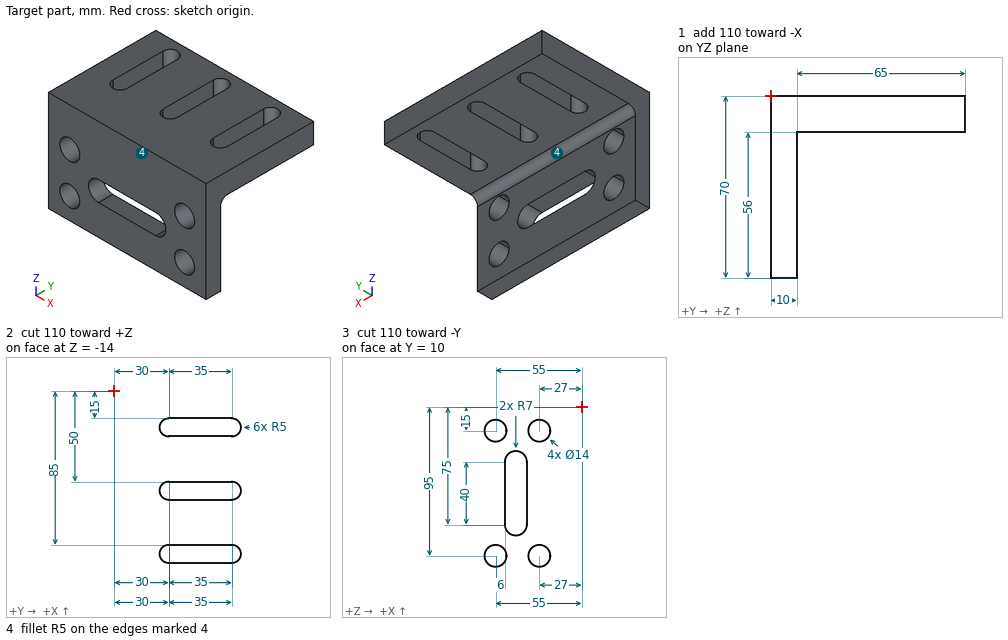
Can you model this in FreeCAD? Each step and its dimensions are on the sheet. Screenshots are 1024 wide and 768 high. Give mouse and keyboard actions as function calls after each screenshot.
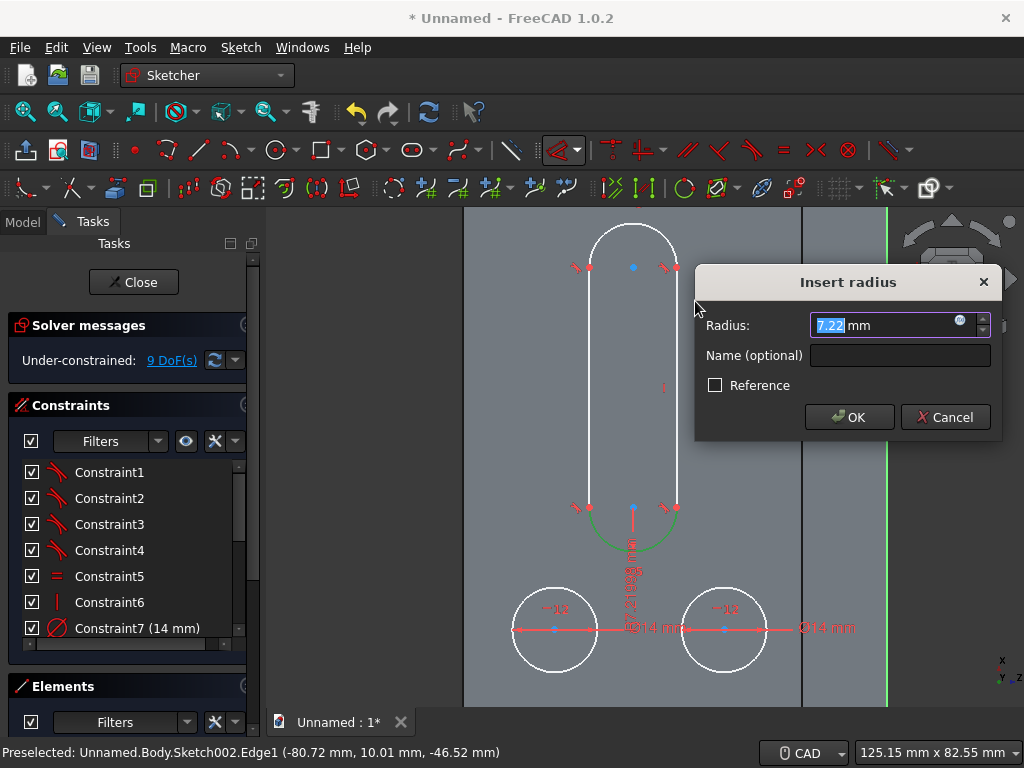
text(7)
key(Return)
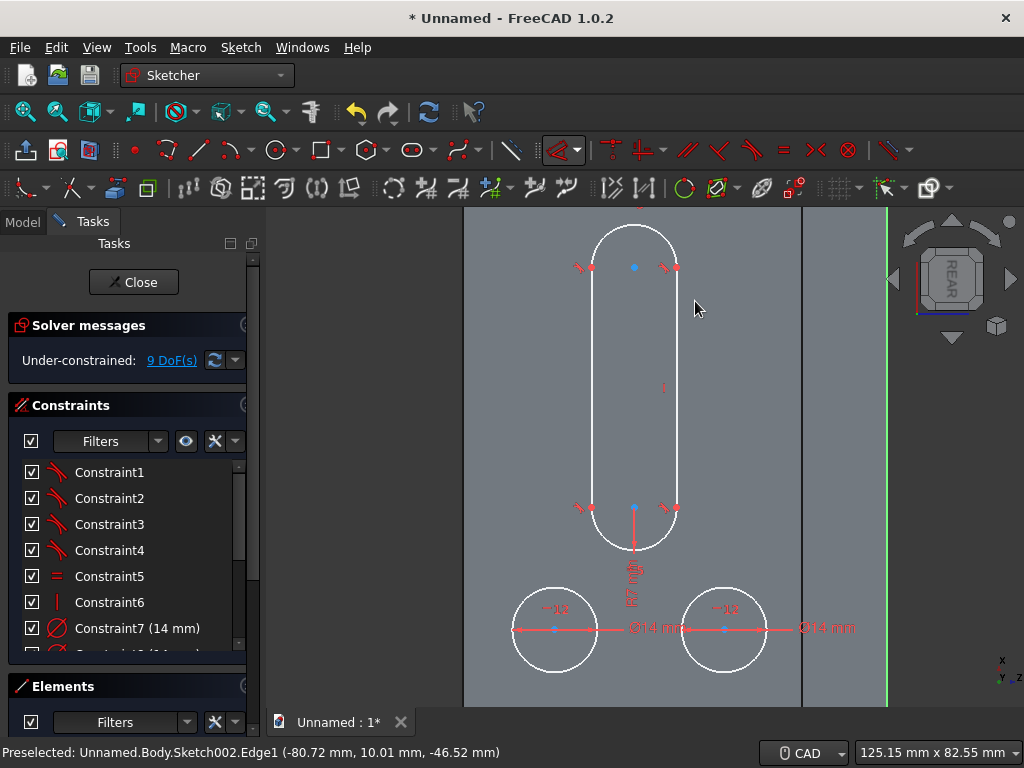
click(592, 436)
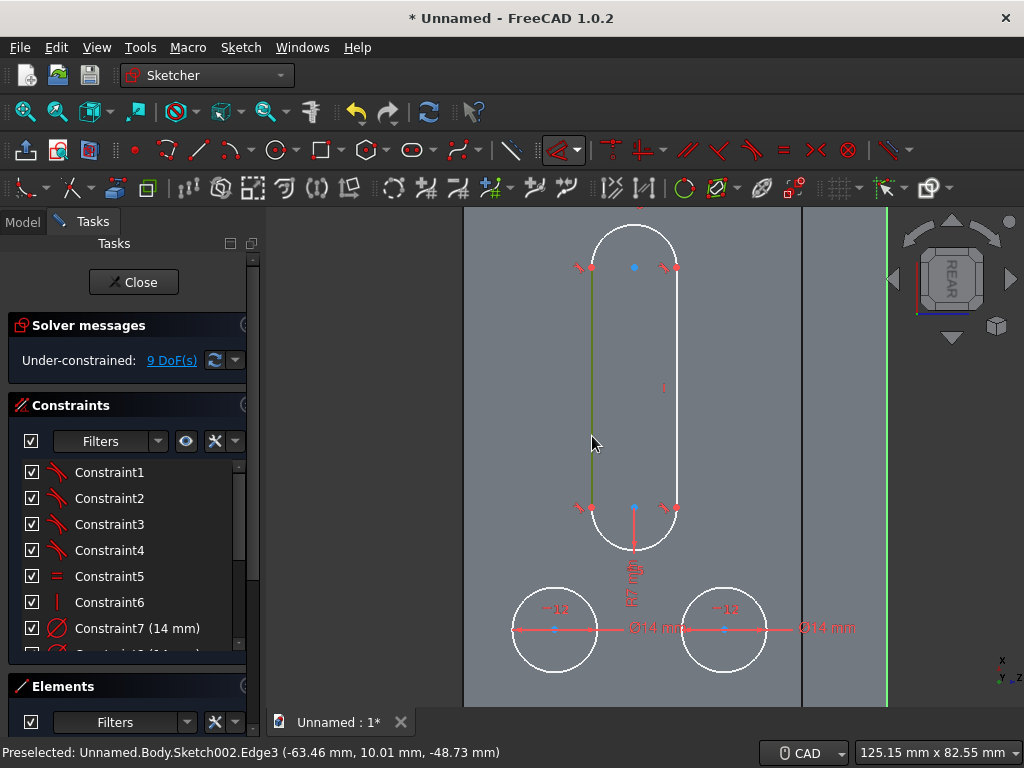
key(i)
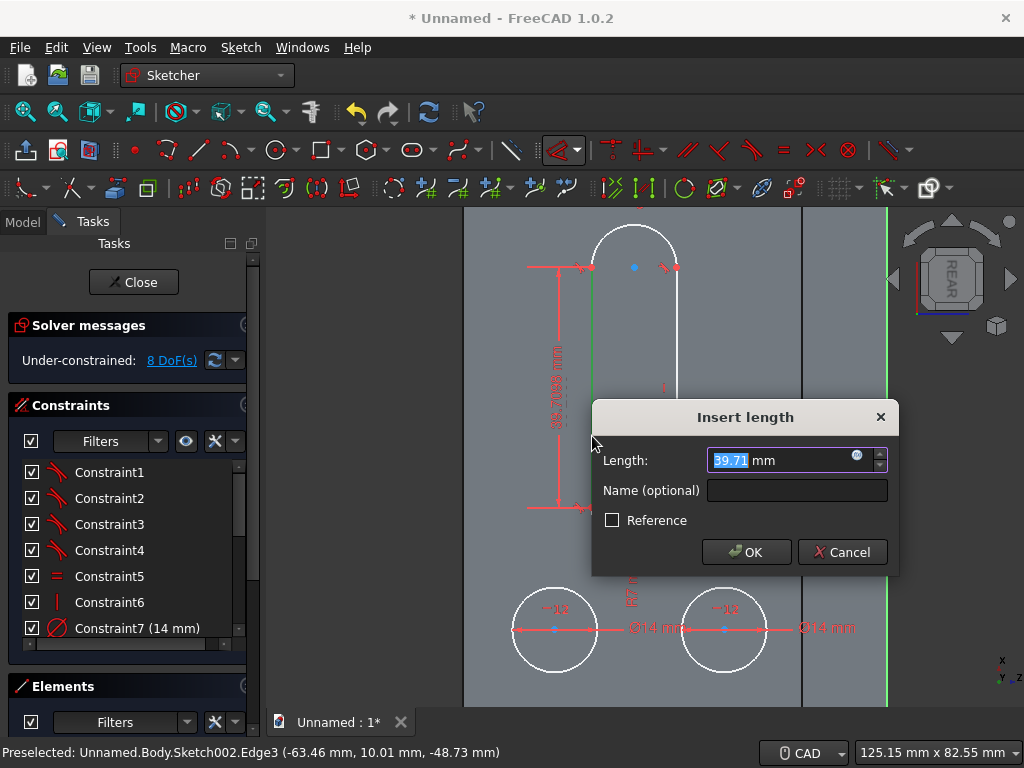
text(40)
key(Return)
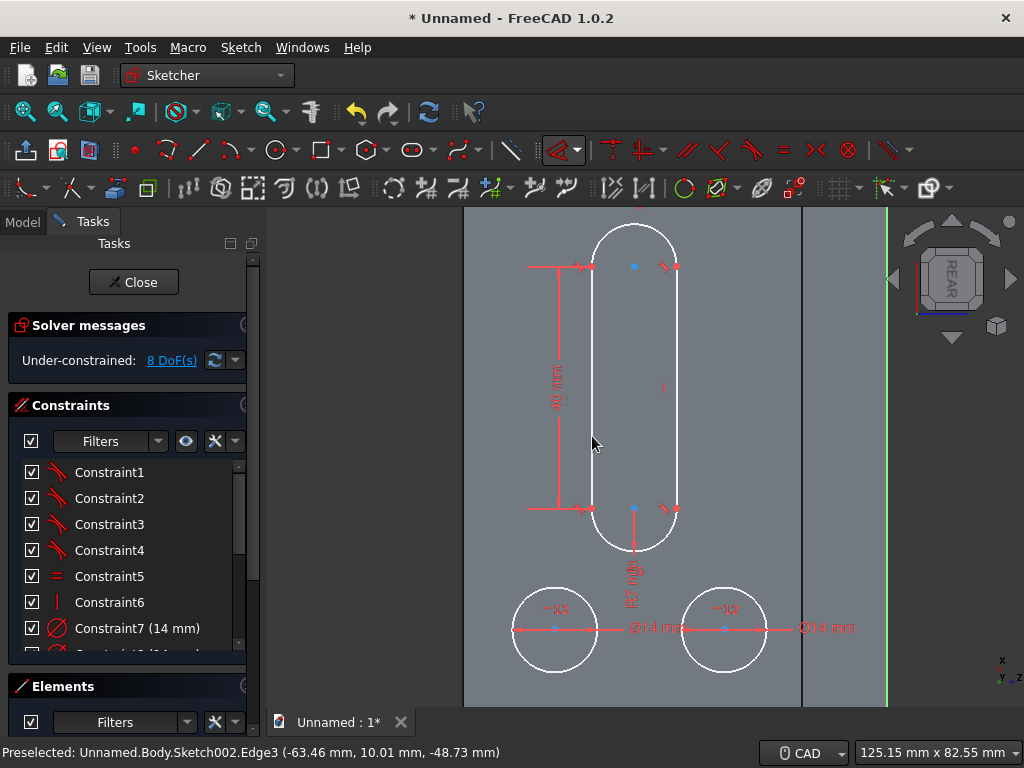
click(555, 630)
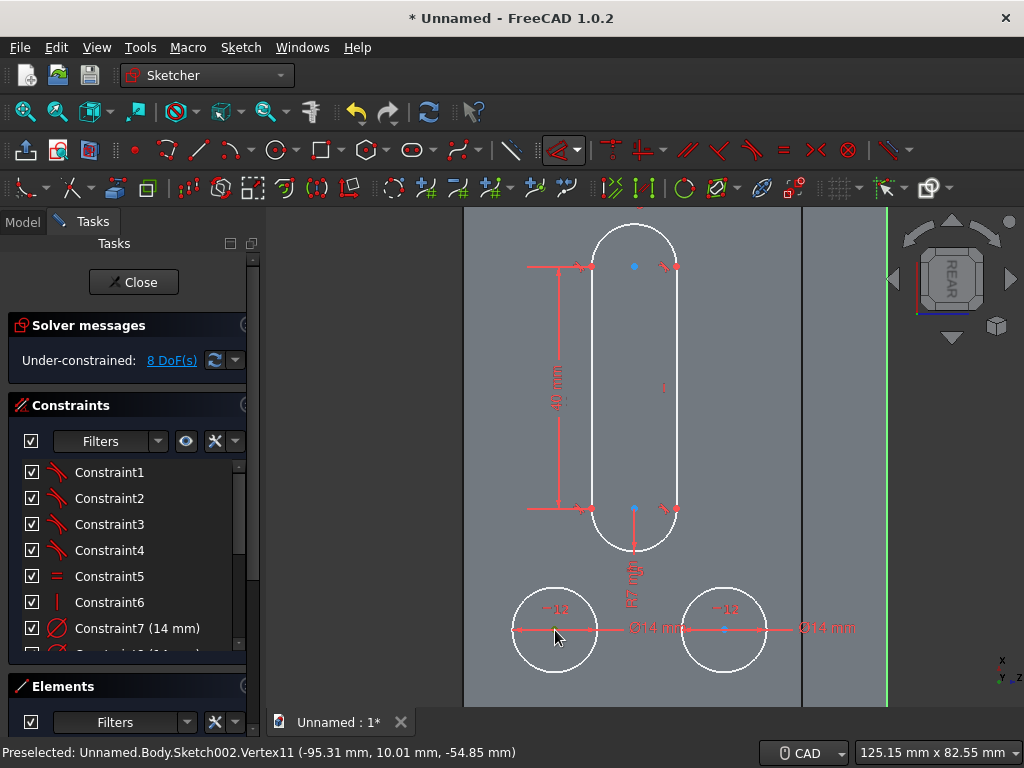
key(l)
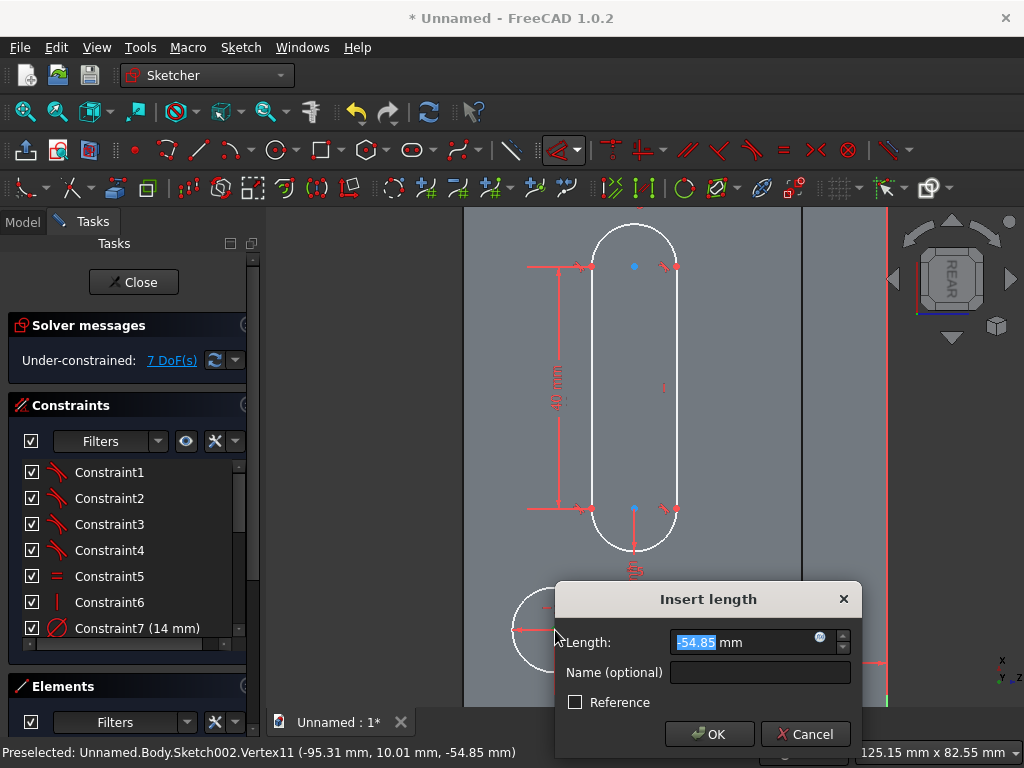
text(-55)
key(Return)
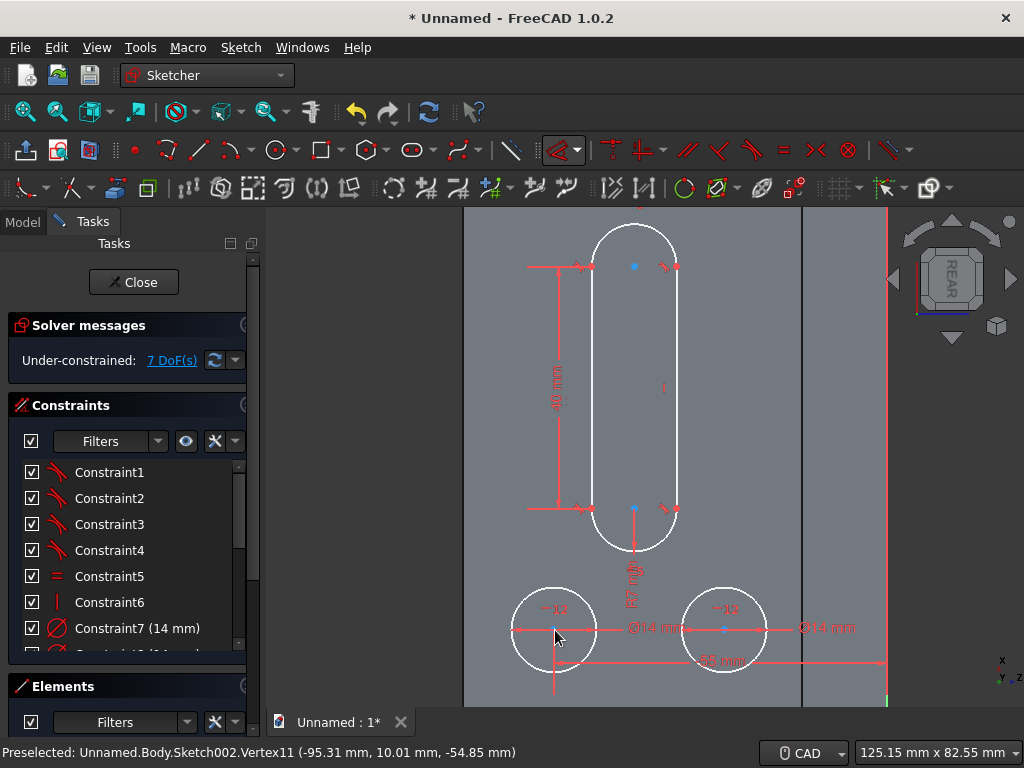
click(554, 630)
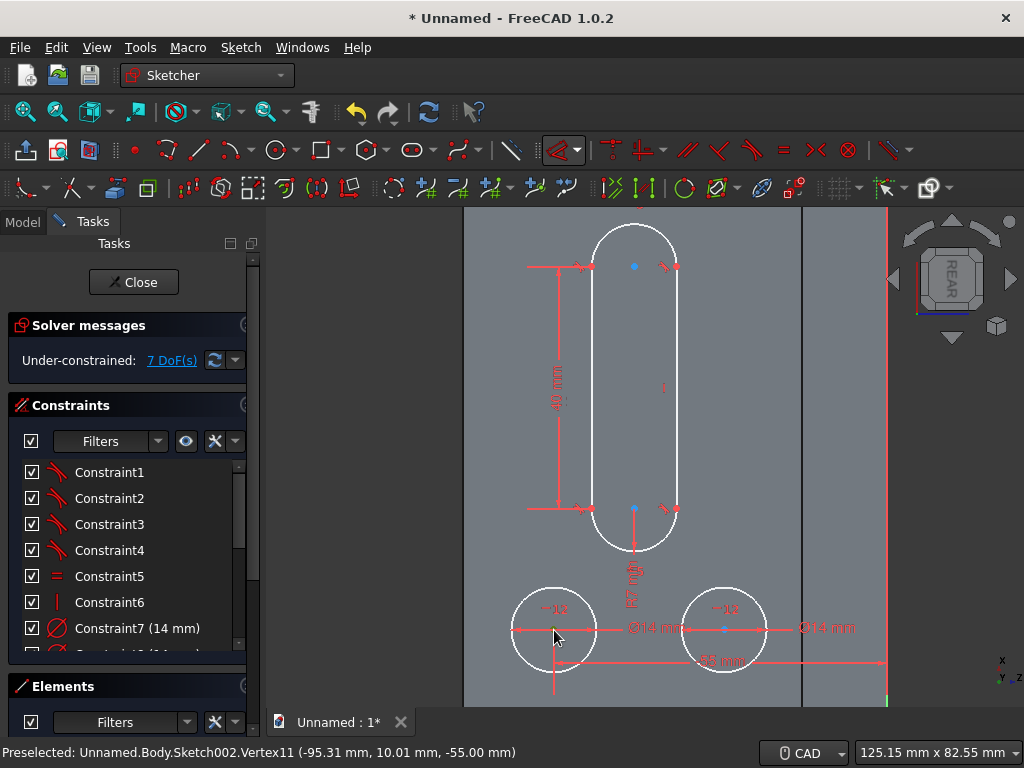
key(i)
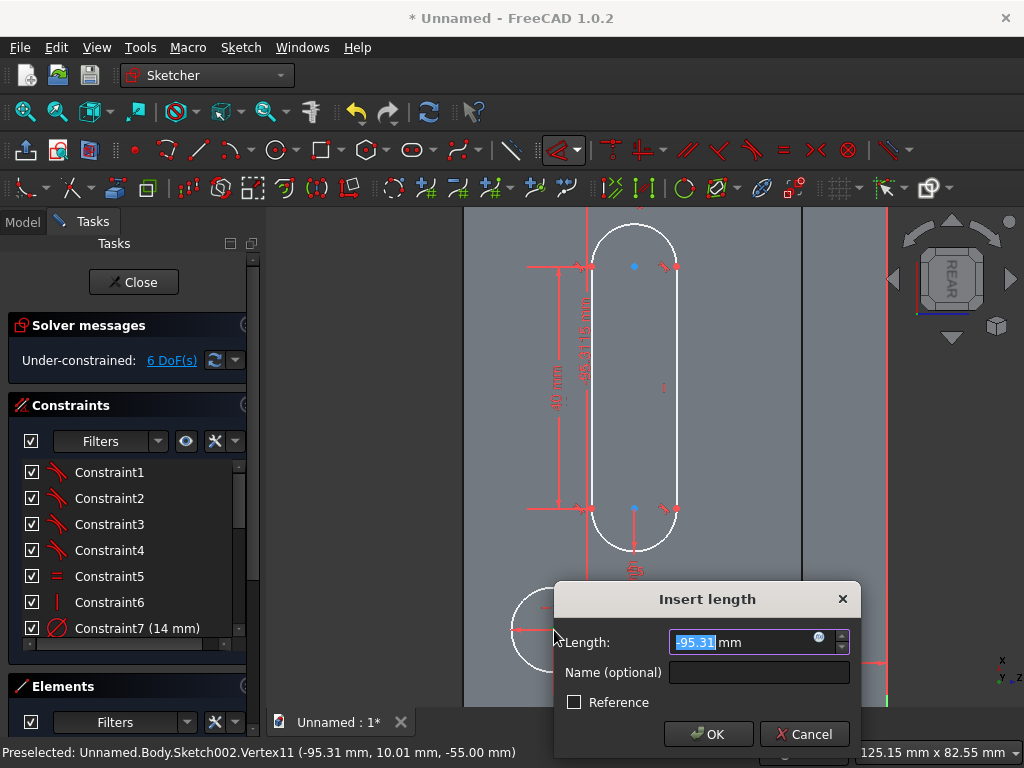
text(-95)
key(Return)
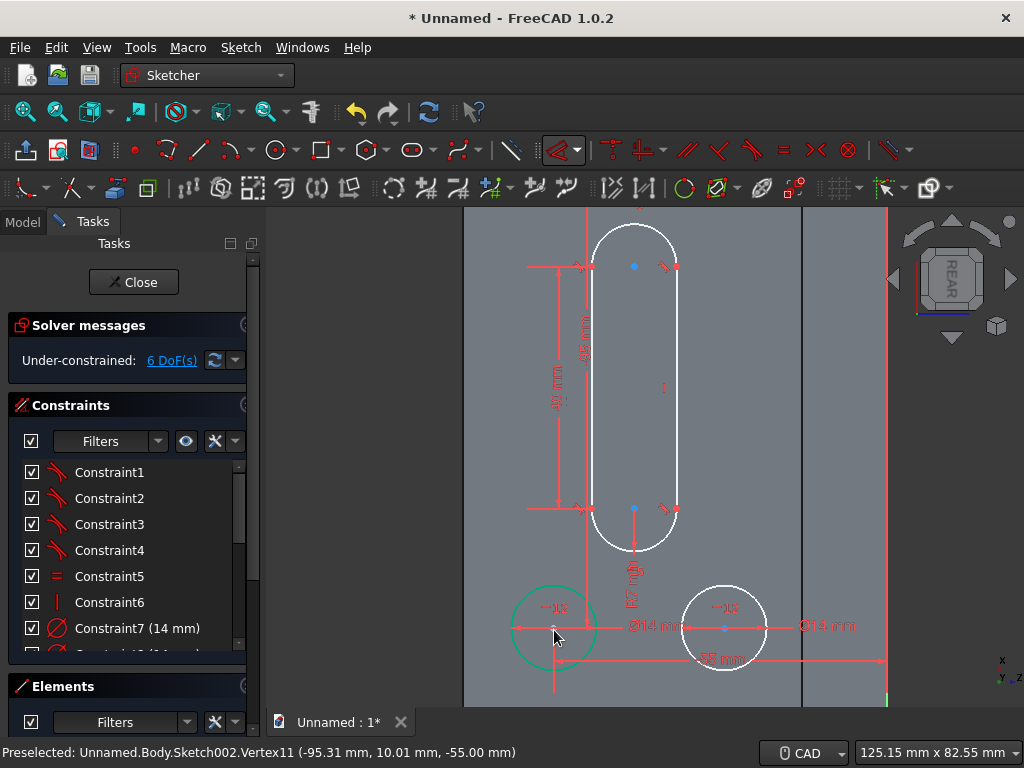
scroll(427, 573, down, 3)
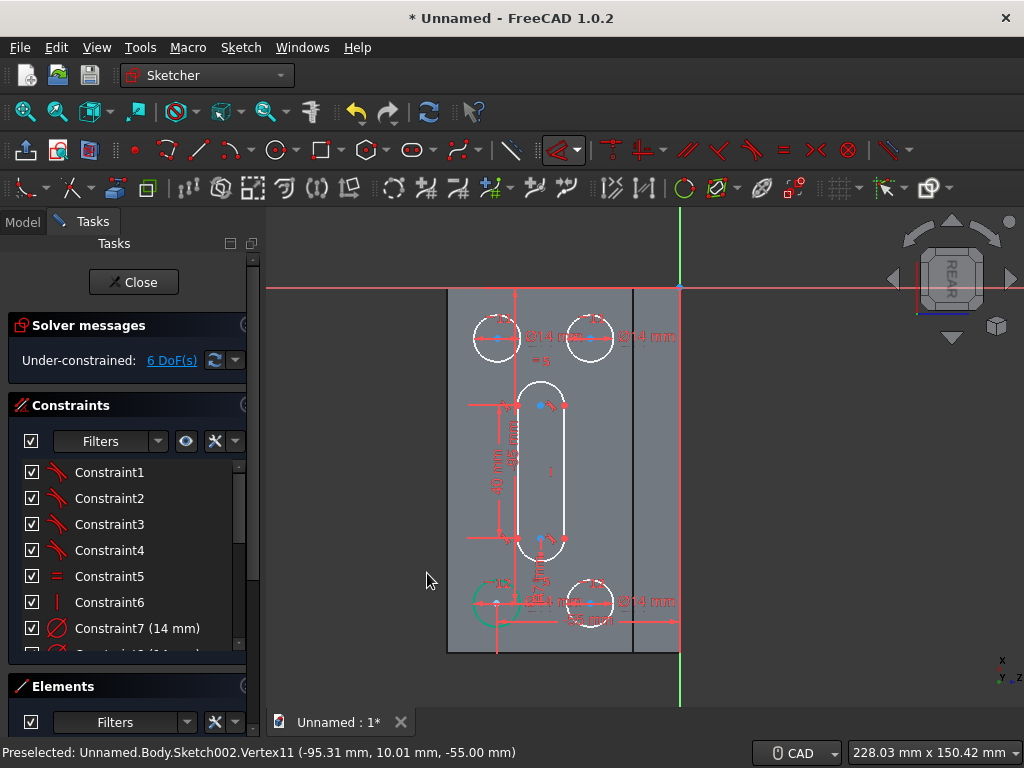
click(497, 339)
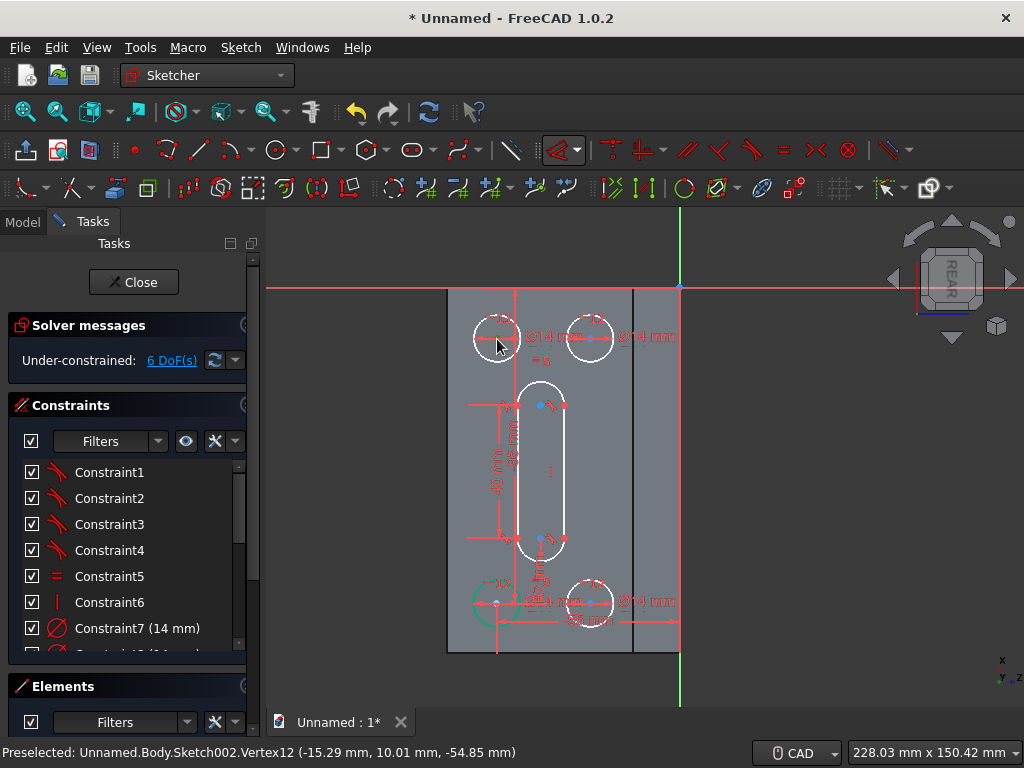
key(l)